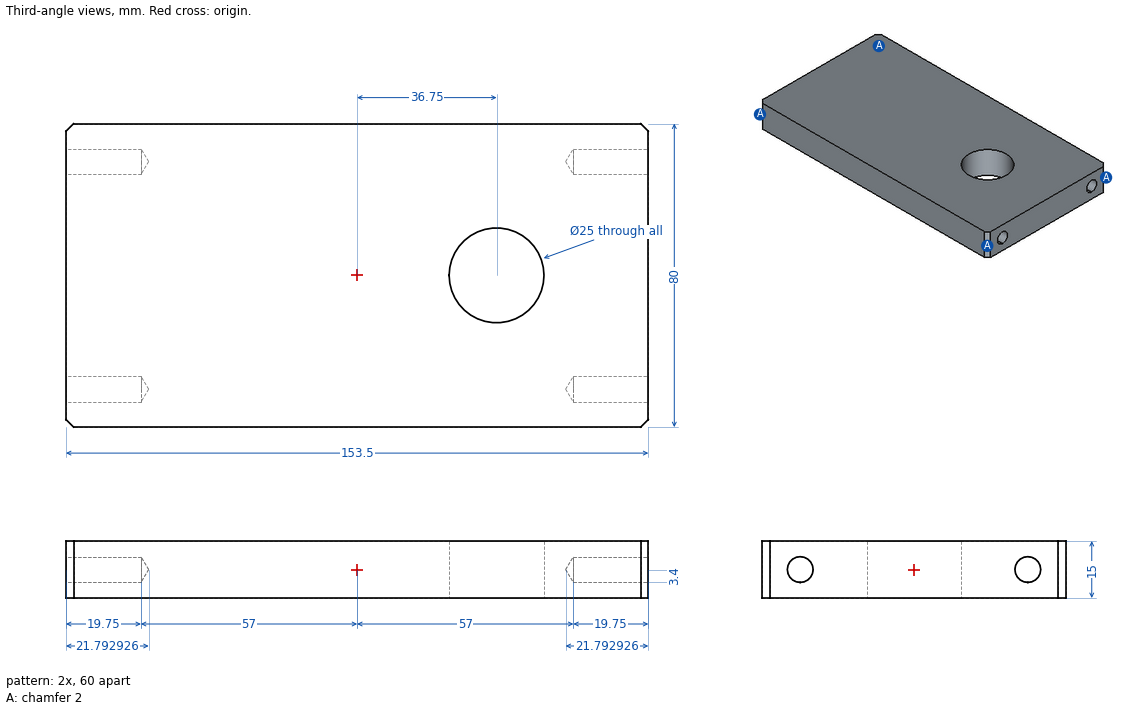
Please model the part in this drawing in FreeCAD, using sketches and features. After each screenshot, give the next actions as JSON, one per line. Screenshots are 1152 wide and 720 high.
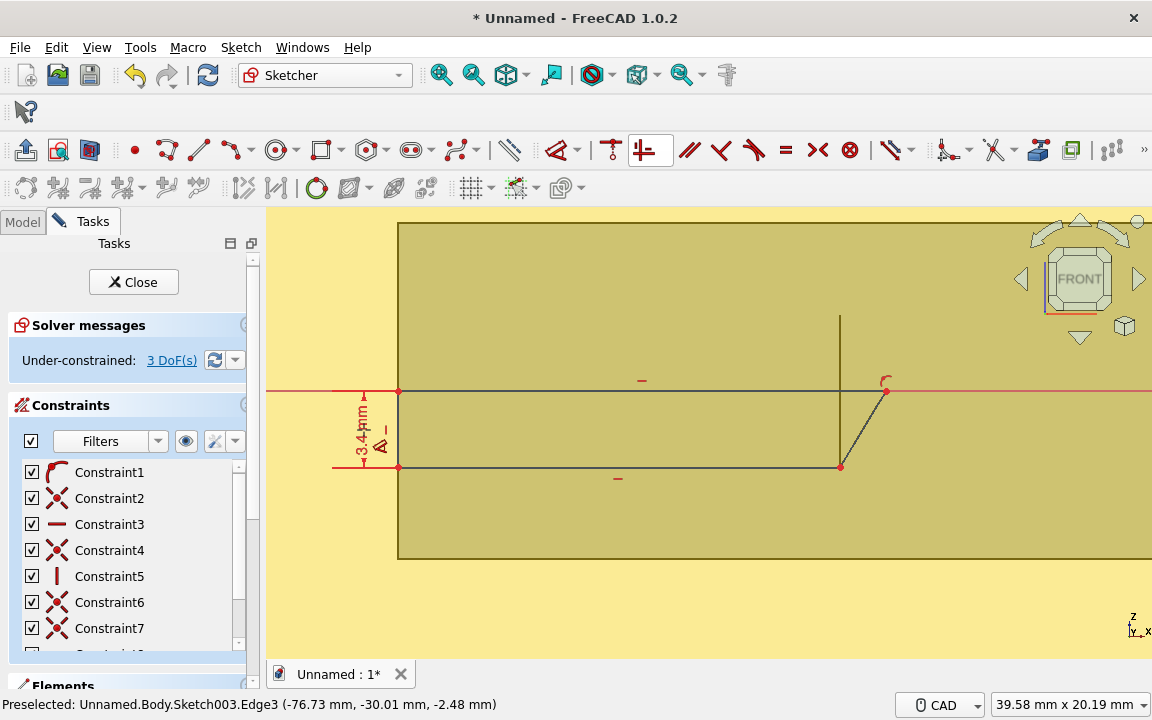
{"action": "left_click", "coordinate": [840, 468]}
{"action": "left_click", "coordinate": [913, 357]}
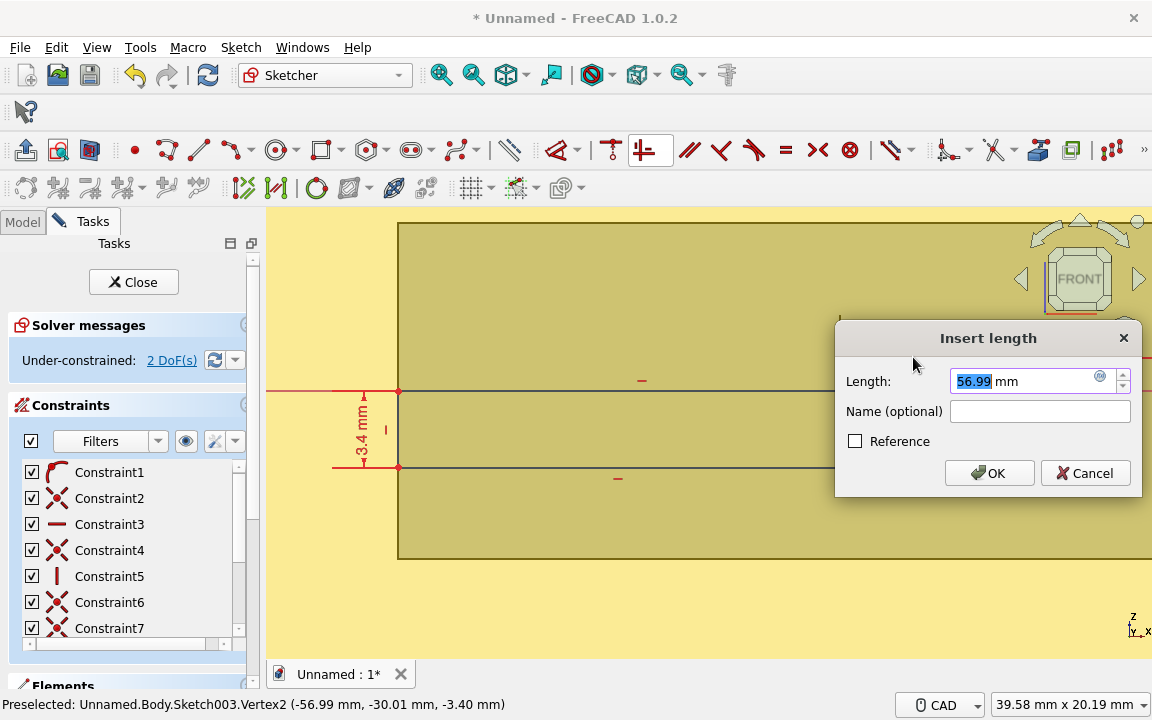
{"action": "type", "text": "57"}
{"action": "key", "text": "Return"}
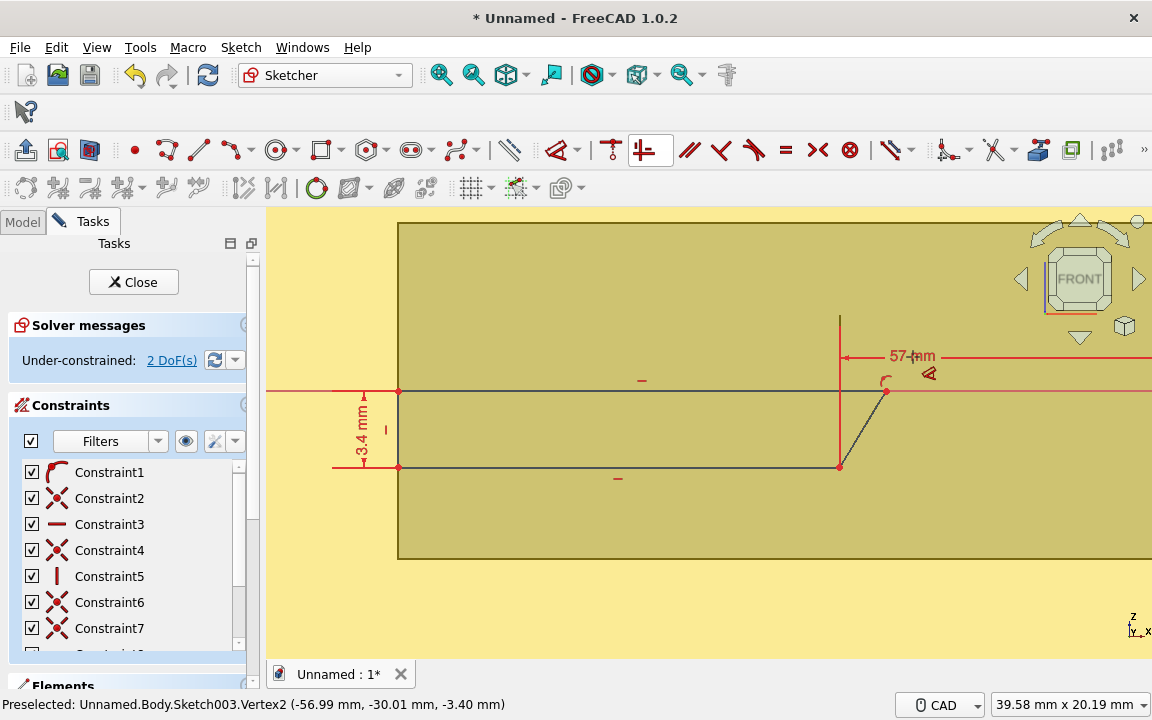
{"action": "left_click", "coordinate": [707, 468]}
{"action": "left_click", "coordinate": [619, 502]}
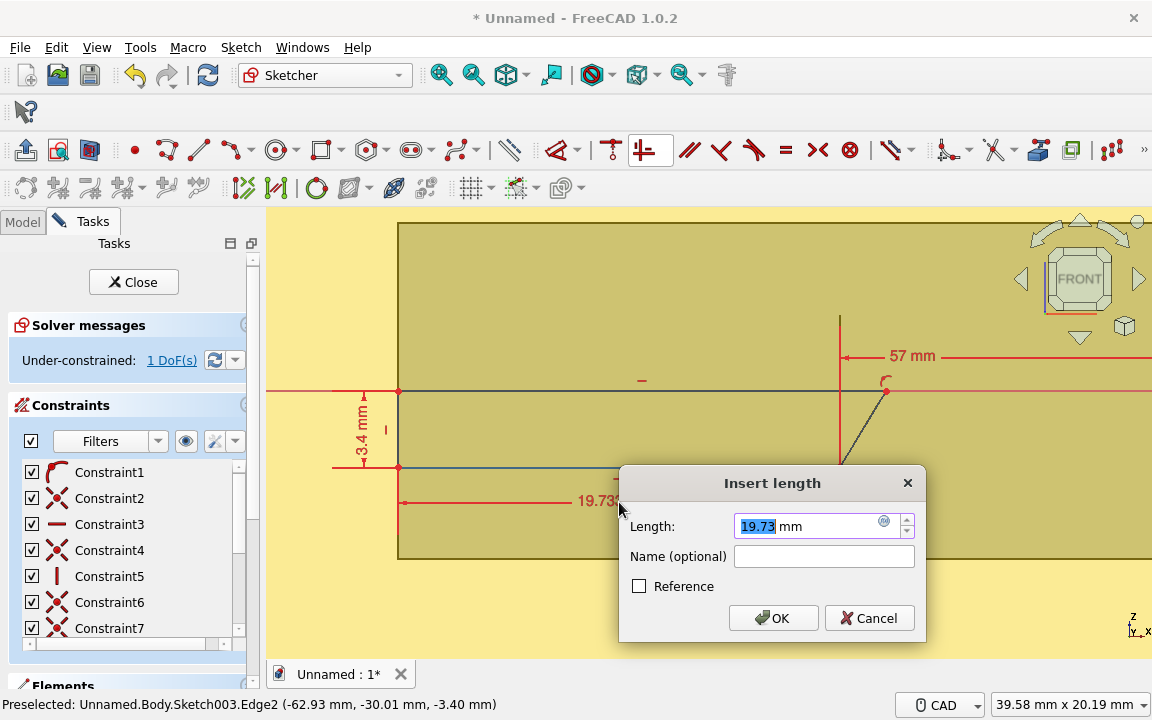
{"action": "type", "text": "19.75"}
{"action": "key", "text": "Return"}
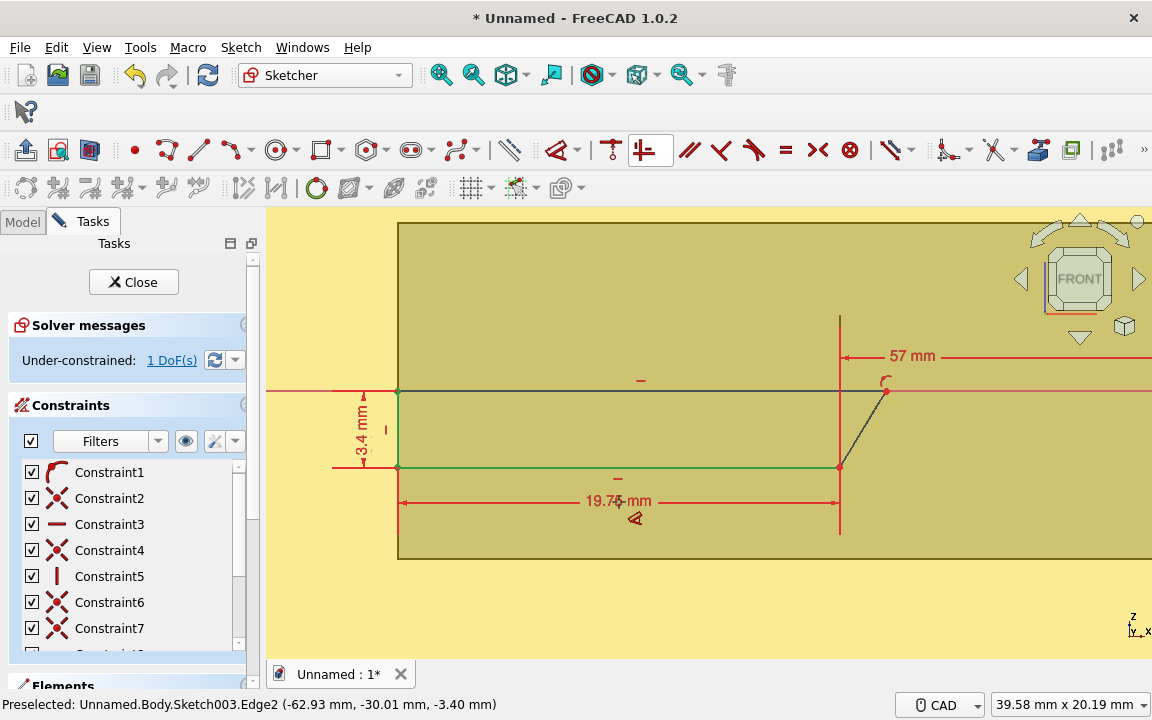
{"action": "left_click", "coordinate": [544, 391]}
{"action": "left_click", "coordinate": [642, 357]}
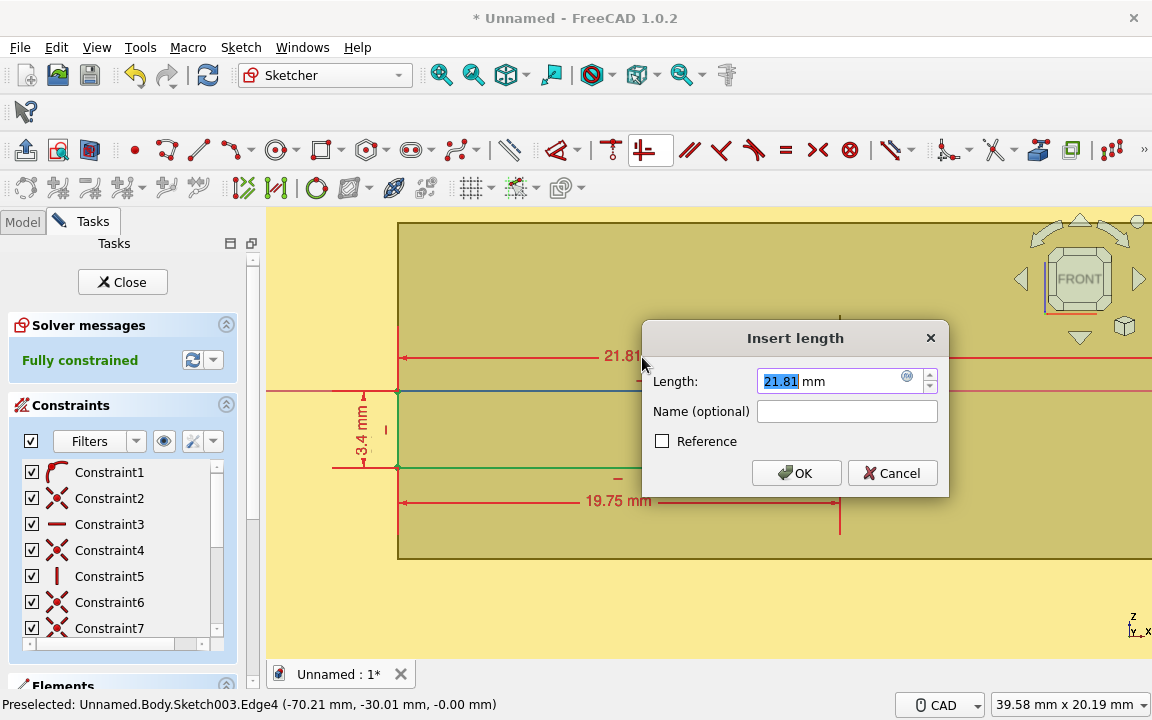
{"action": "type", "text": "21.792926"}
{"action": "key", "text": "Return"}
{"action": "key", "text": "Escape"}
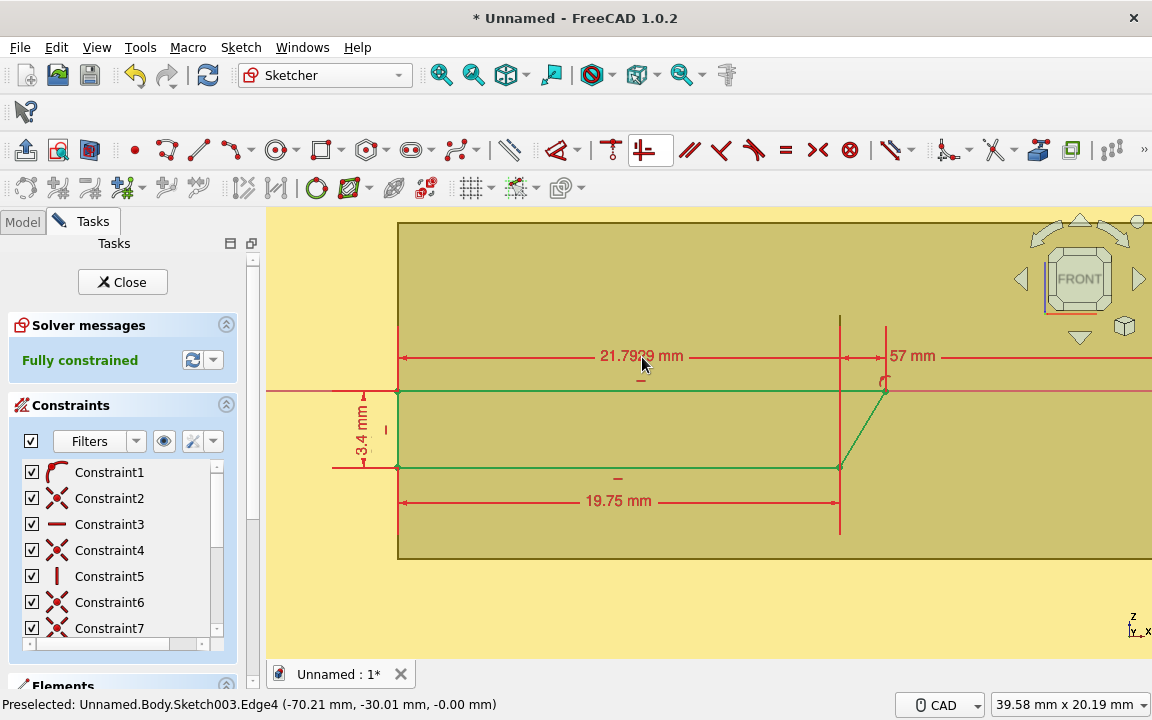
{"action": "left_click", "coordinate": [123, 282]}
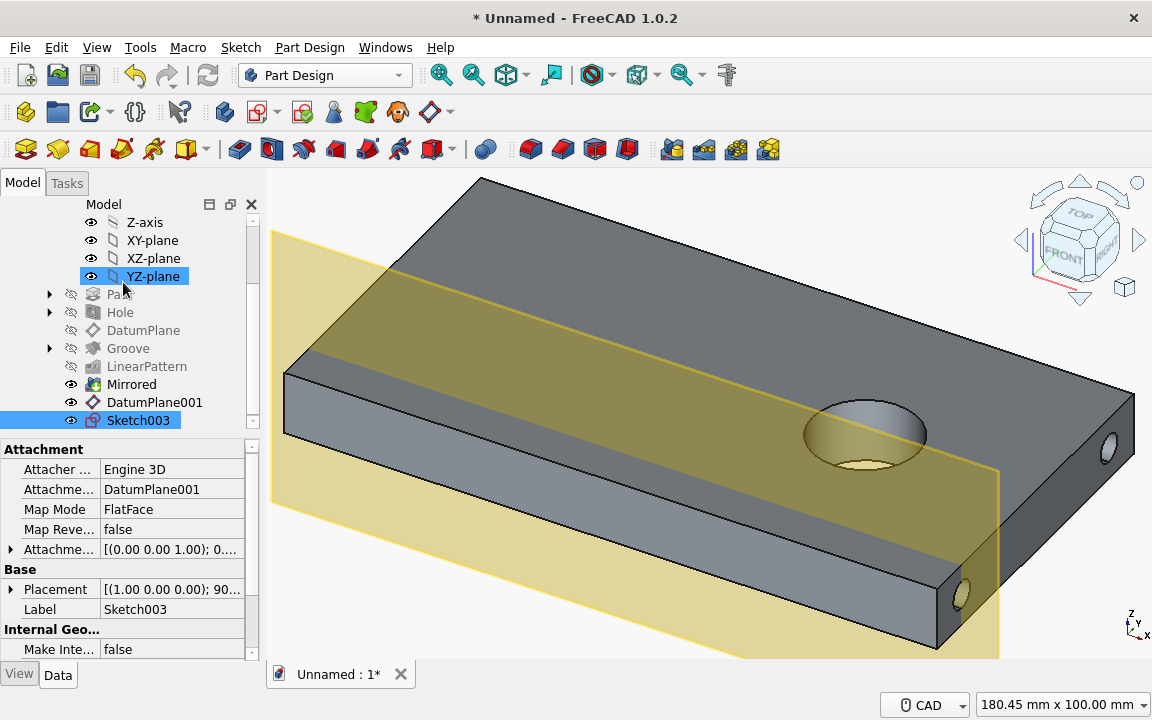
{"action": "left_click", "coordinate": [304, 150]}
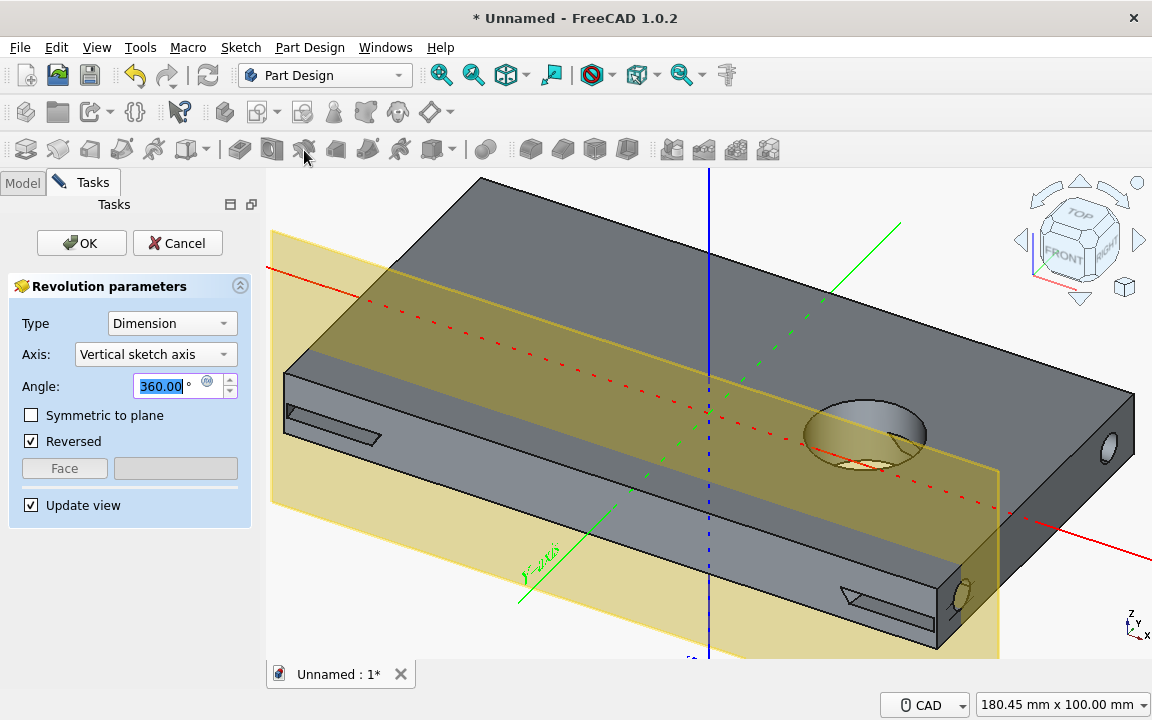
{"action": "left_click", "coordinate": [156, 354]}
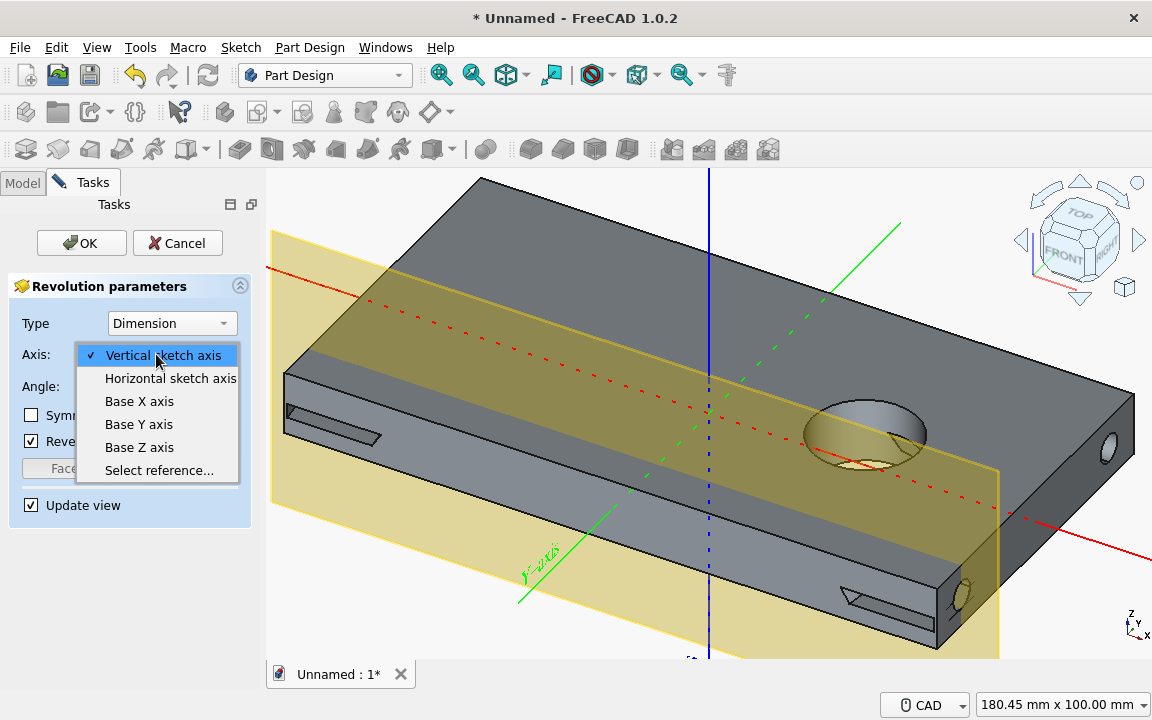
{"action": "left_click", "coordinate": [156, 378]}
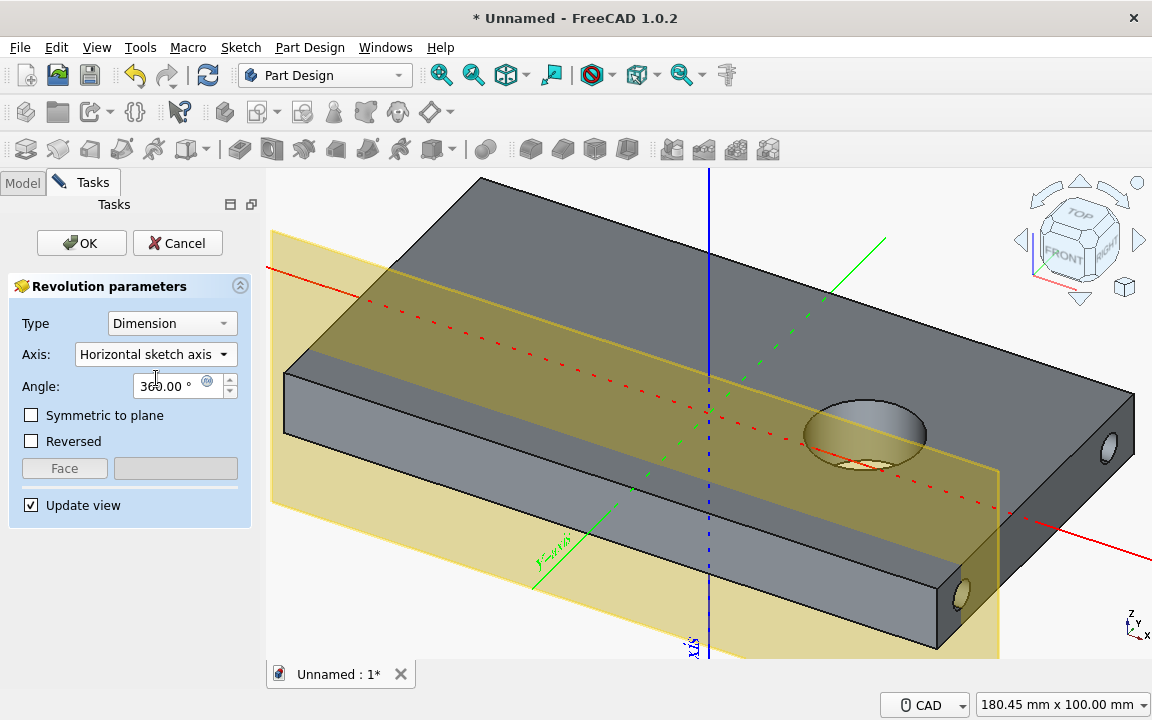
{"action": "left_click", "coordinate": [82, 243]}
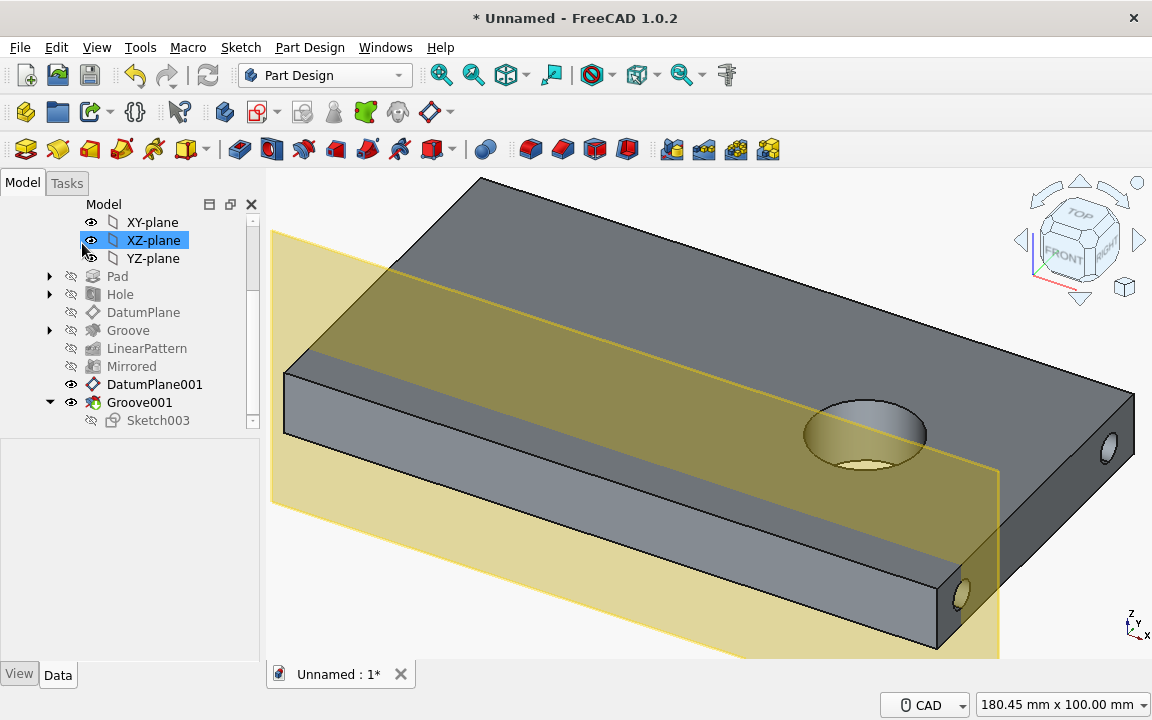
{"action": "left_click", "coordinate": [116, 384]}
{"action": "key", "text": "space"}